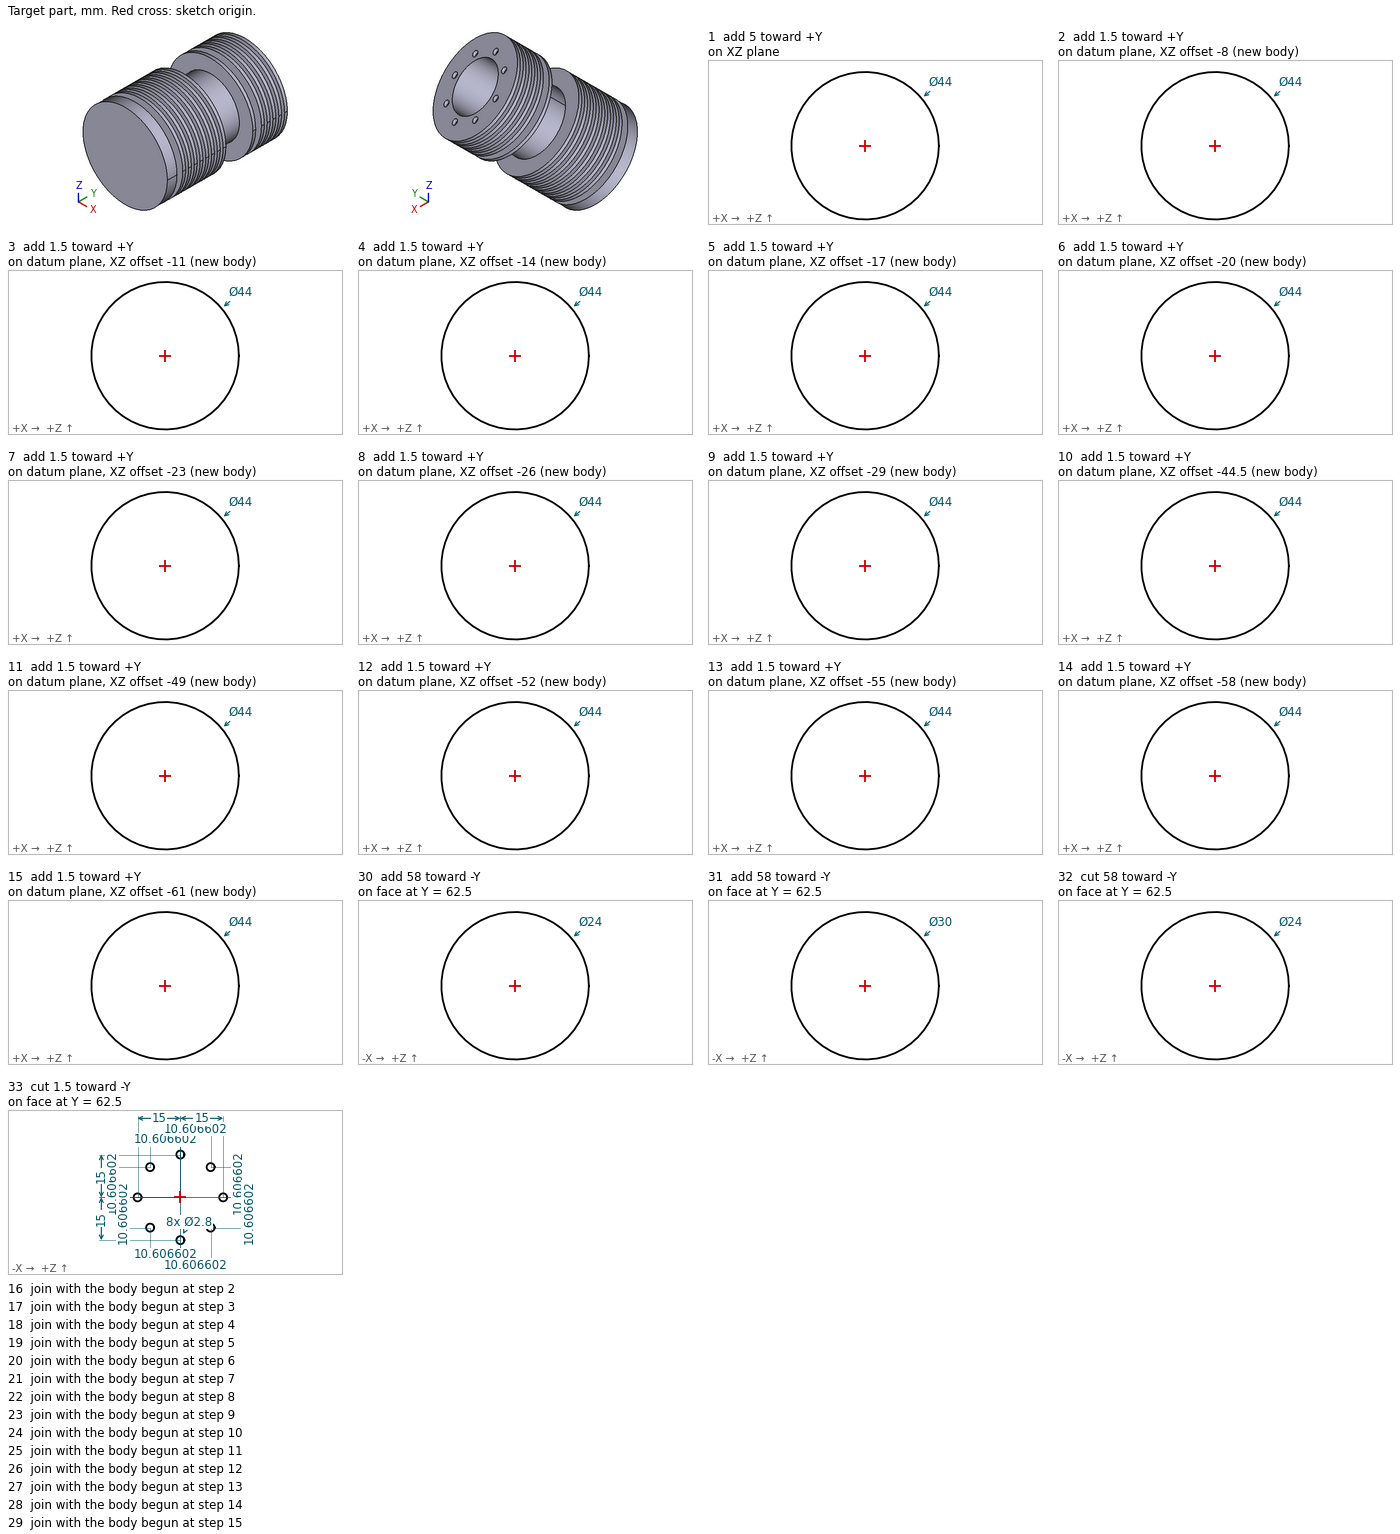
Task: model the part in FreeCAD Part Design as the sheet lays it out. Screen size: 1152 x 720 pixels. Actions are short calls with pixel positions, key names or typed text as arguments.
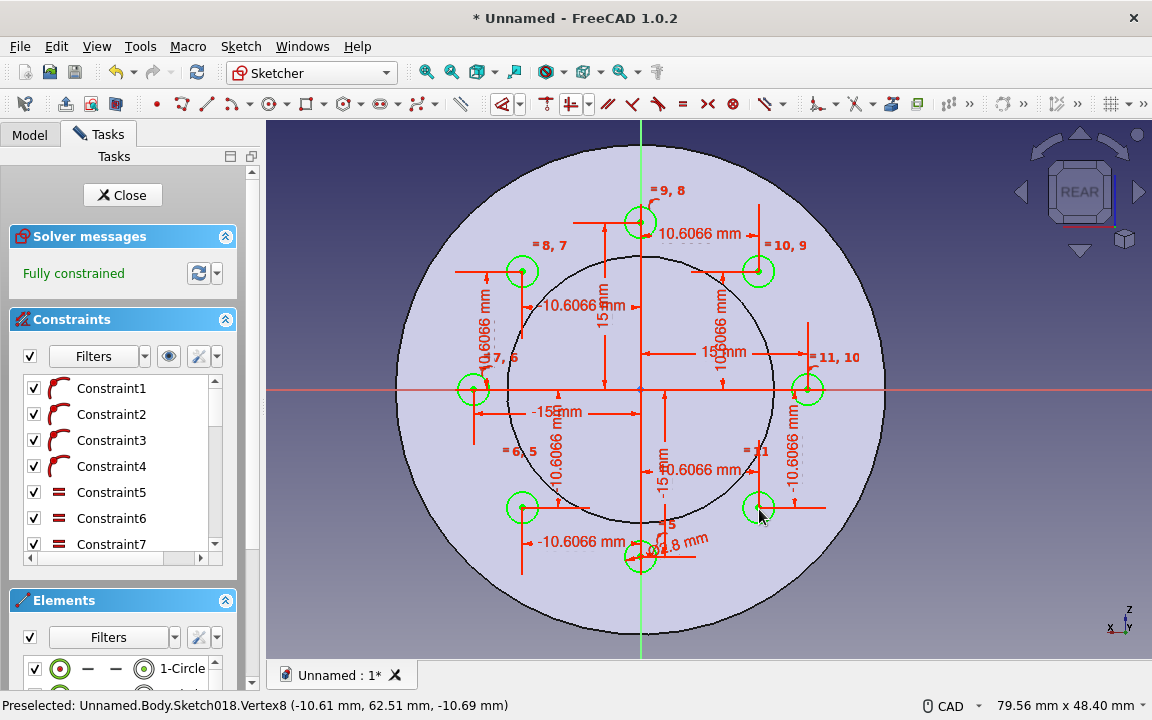
click(123, 195)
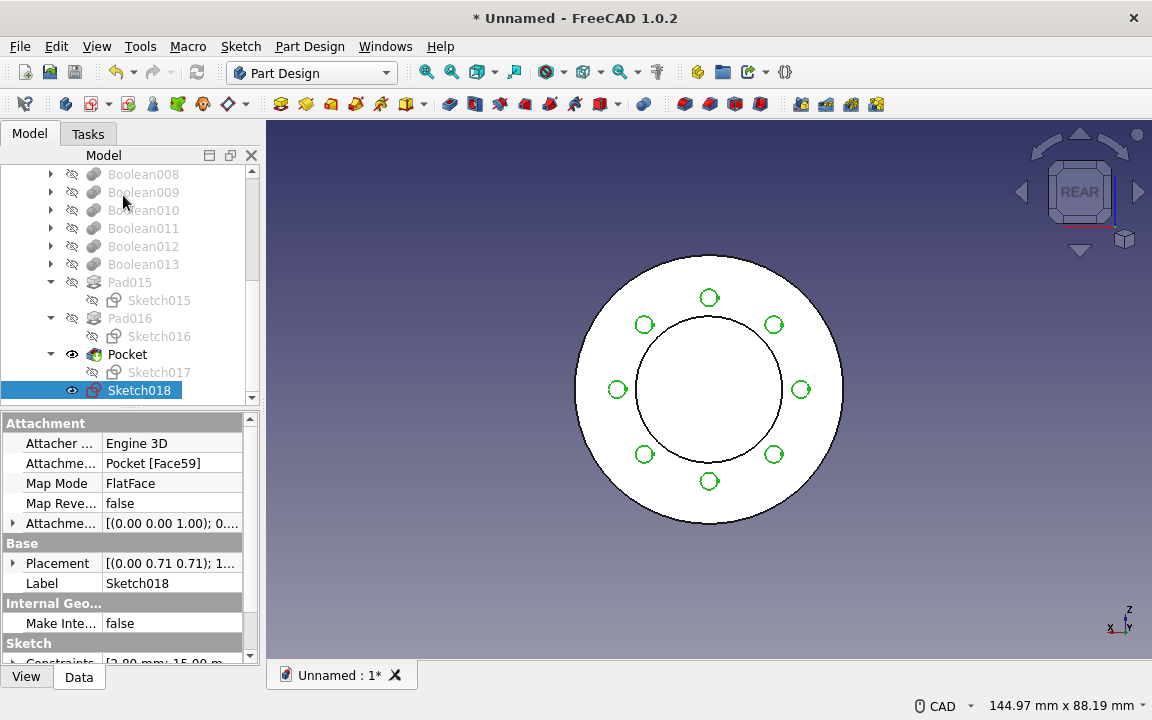
click(450, 104)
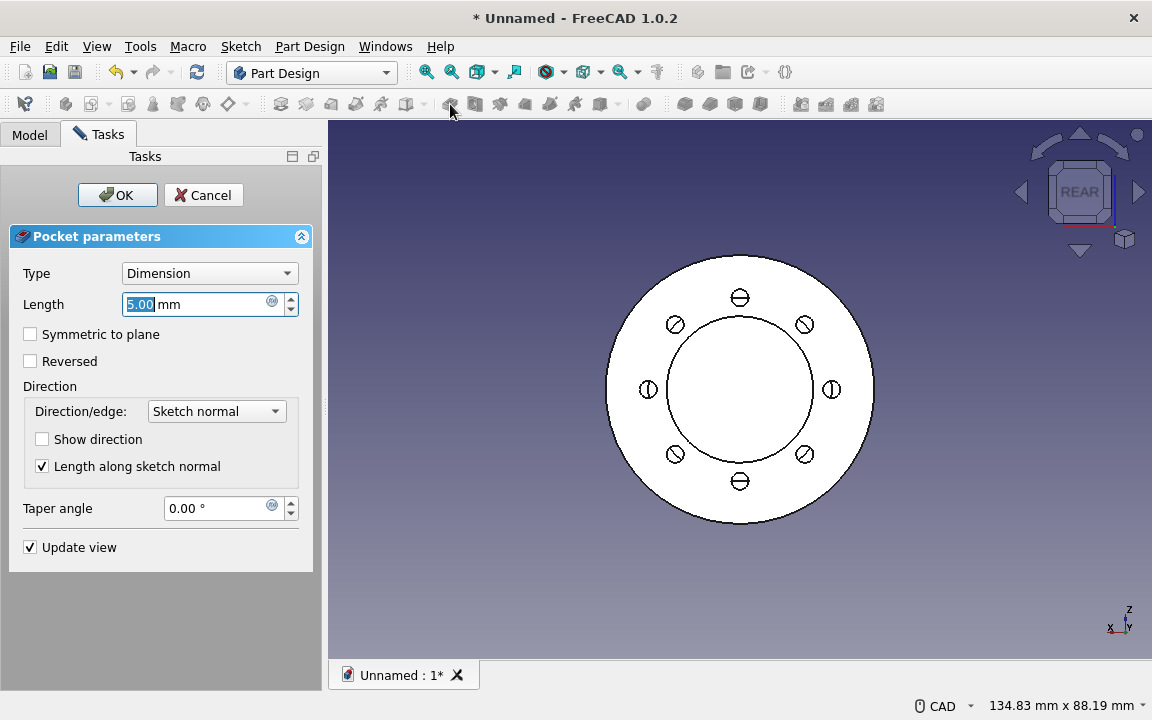
text(1.5)
key(Tab)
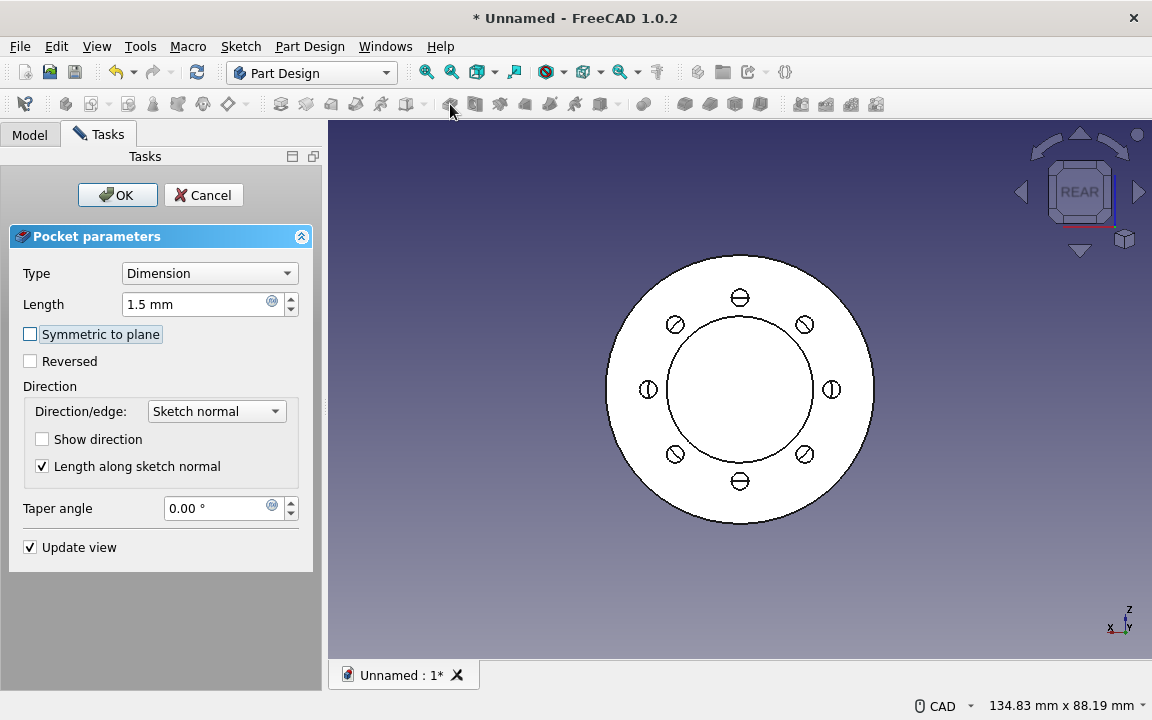
click(118, 195)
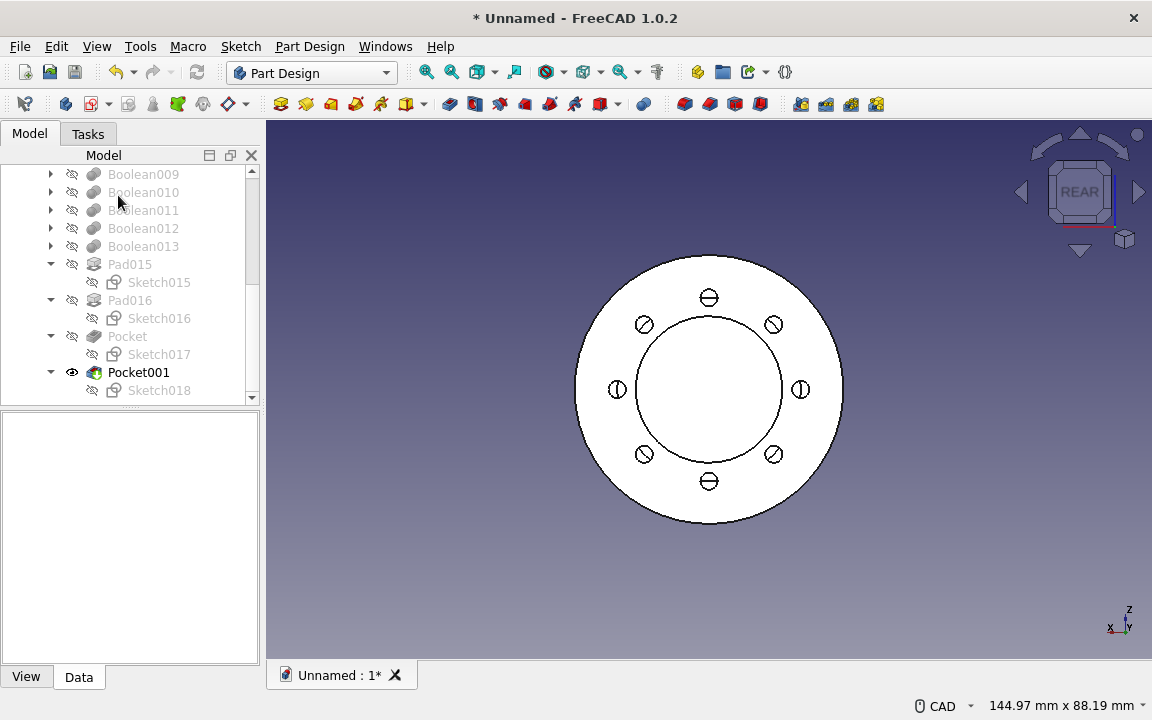
key(0)